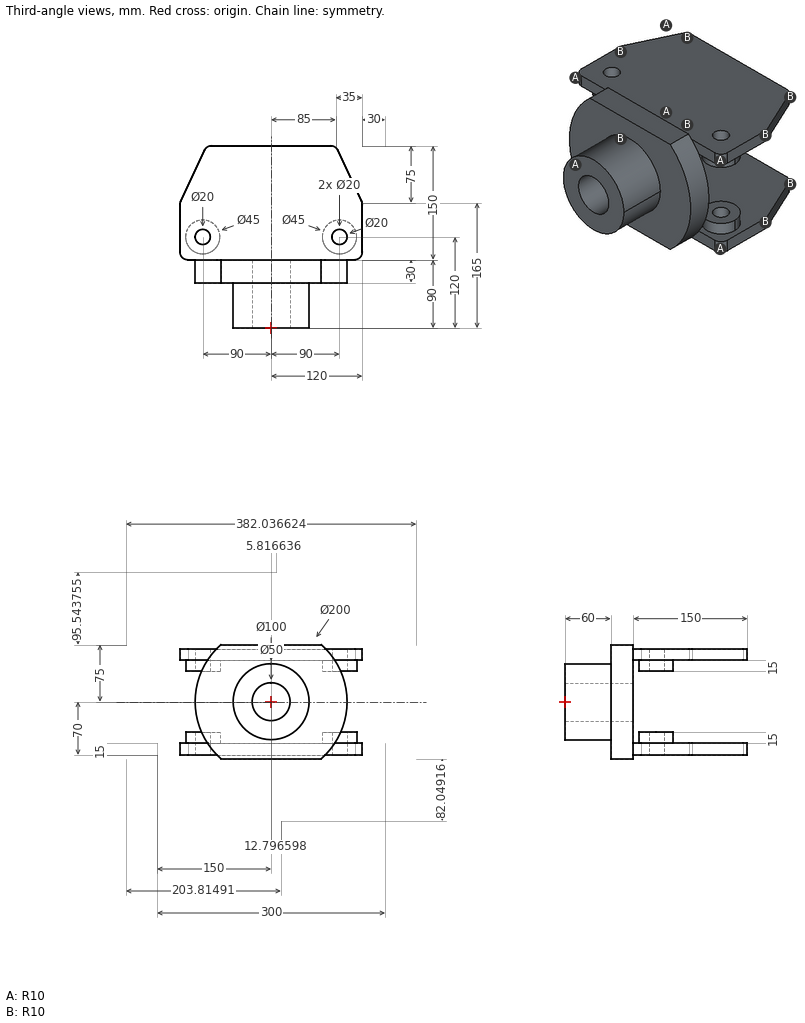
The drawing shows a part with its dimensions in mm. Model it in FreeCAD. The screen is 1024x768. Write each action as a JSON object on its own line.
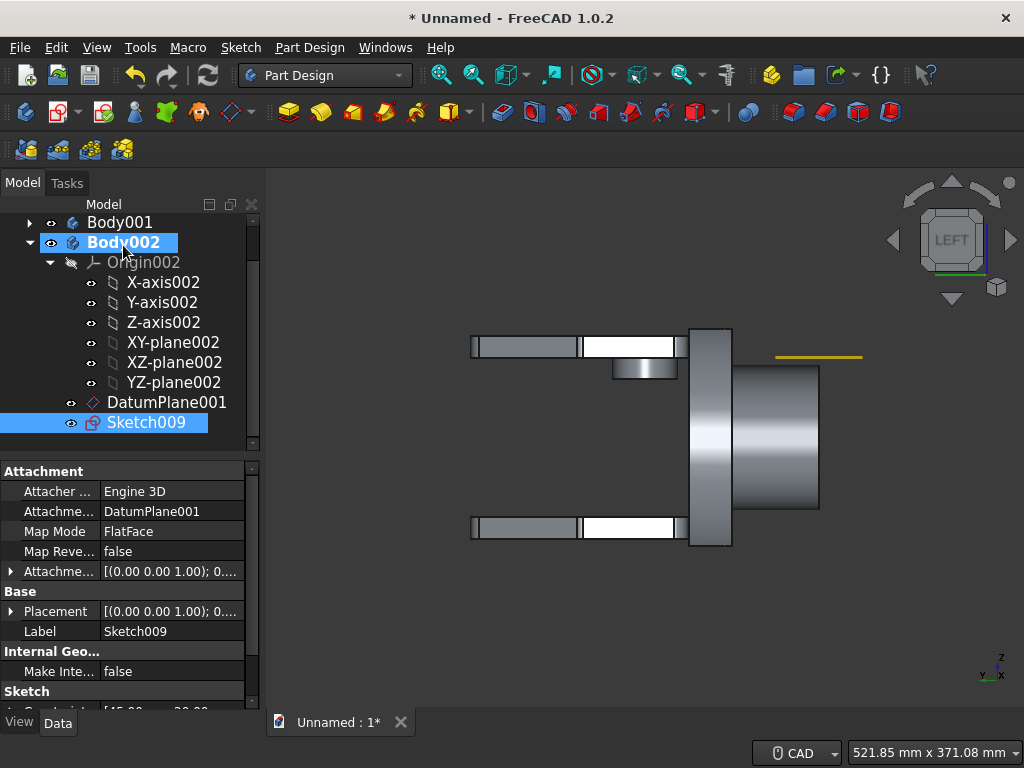
{"action": "left_click", "coordinate": [290, 112]}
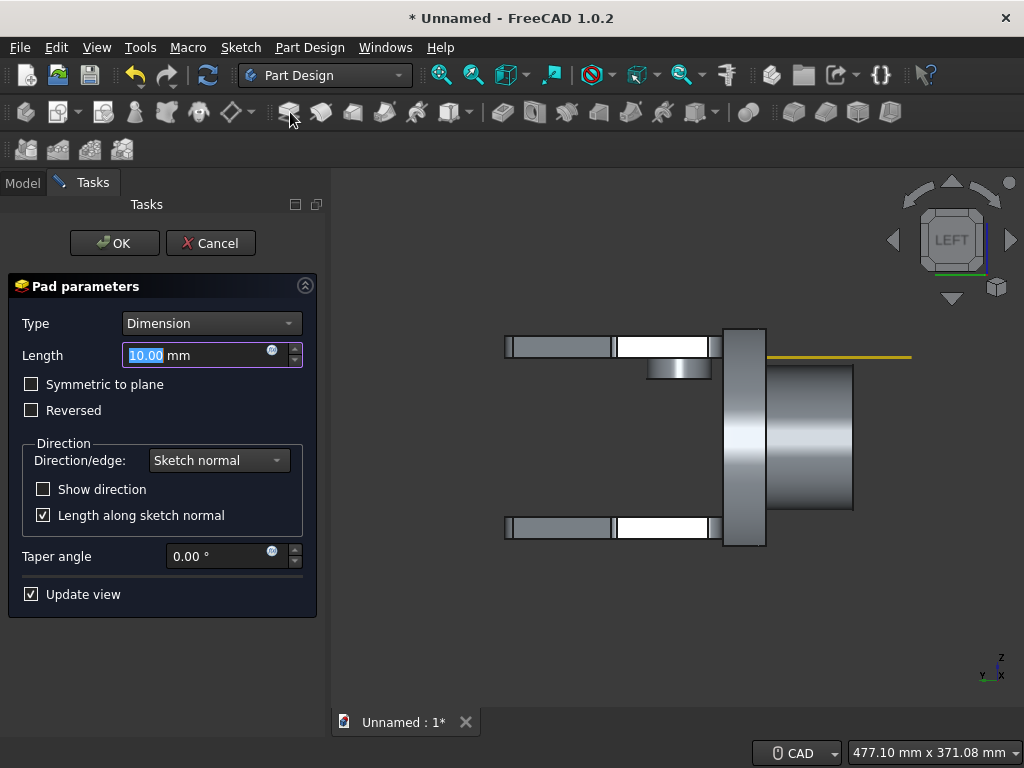
{"action": "type", "text": "15"}
{"action": "key", "text": "Tab"}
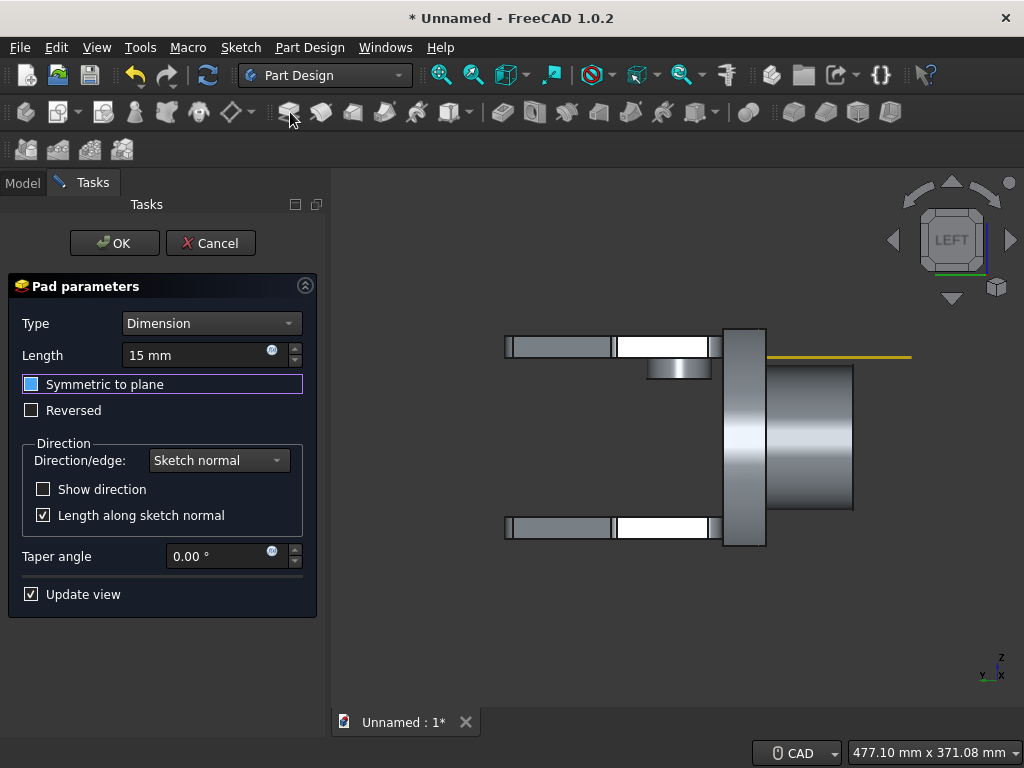
{"action": "left_click", "coordinate": [30, 410]}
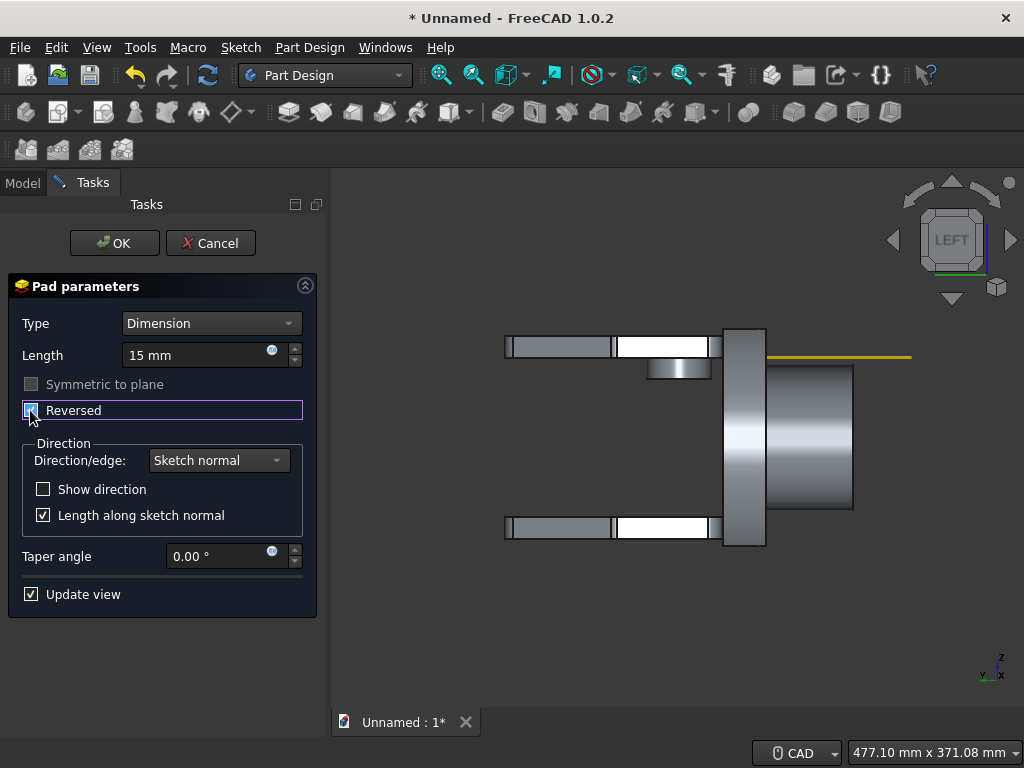
{"action": "left_click", "coordinate": [115, 243]}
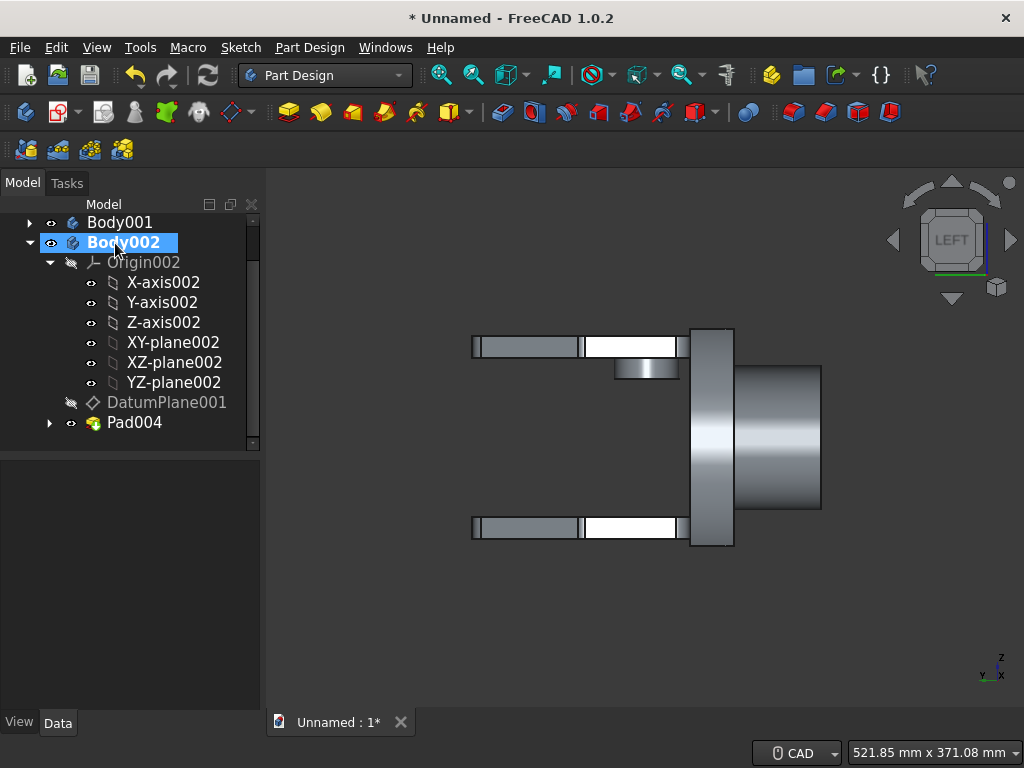
{"action": "left_click", "coordinate": [442, 76]}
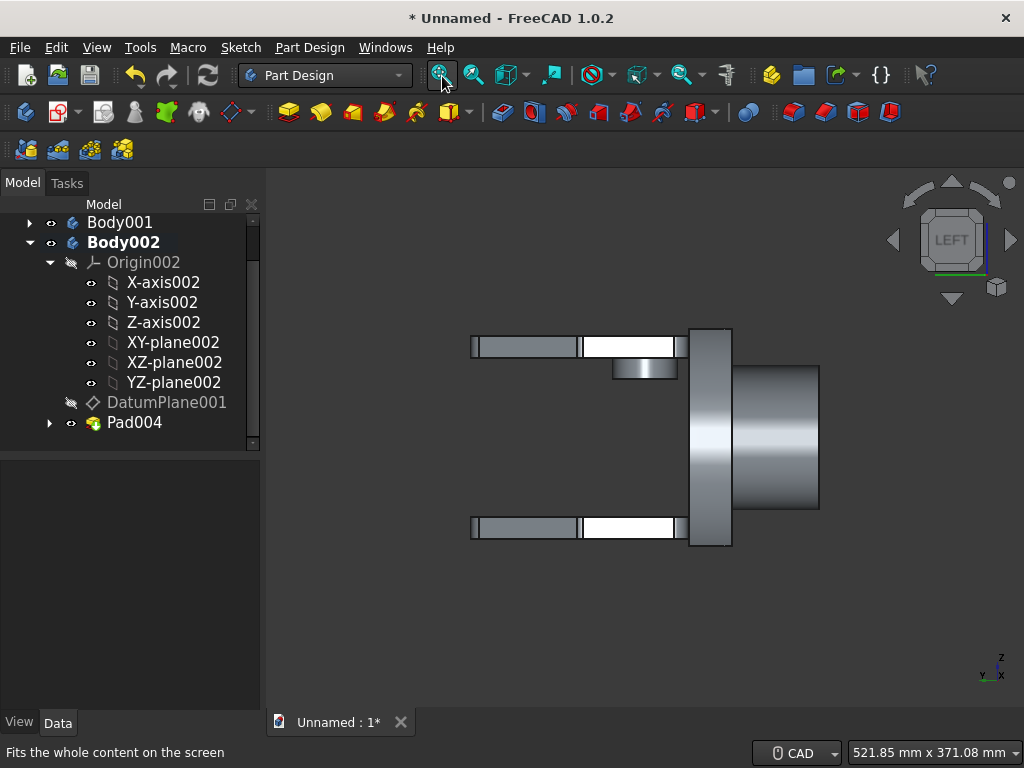
{"action": "left_click", "coordinate": [26, 112]}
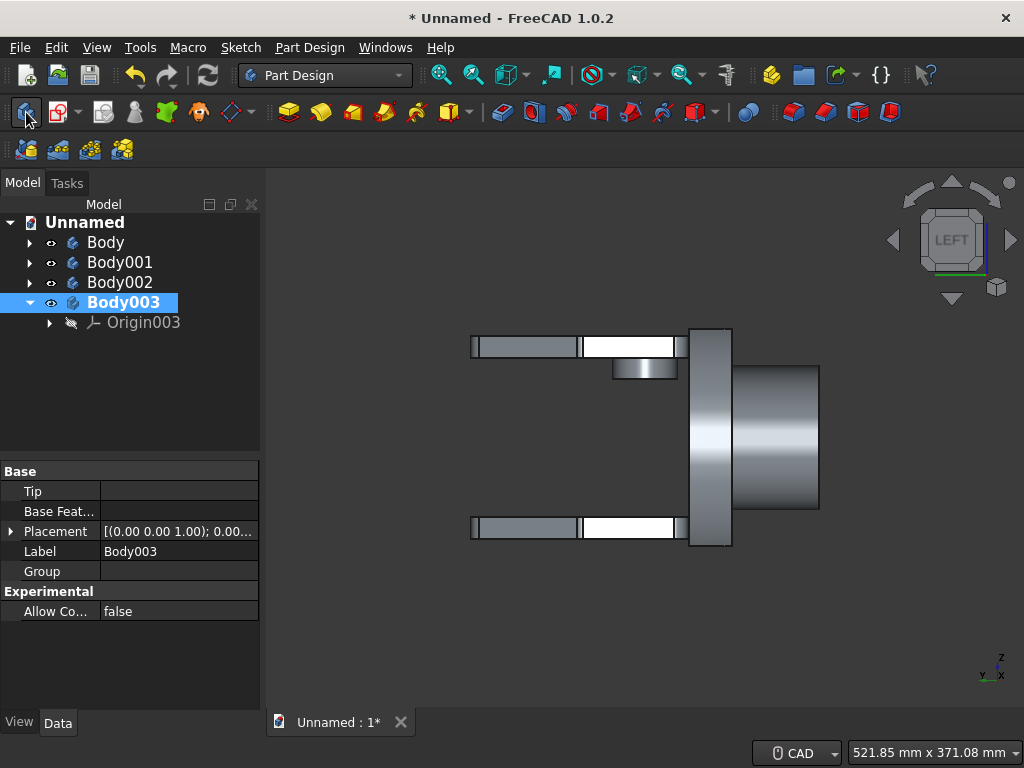
{"action": "left_click", "coordinate": [50, 323]}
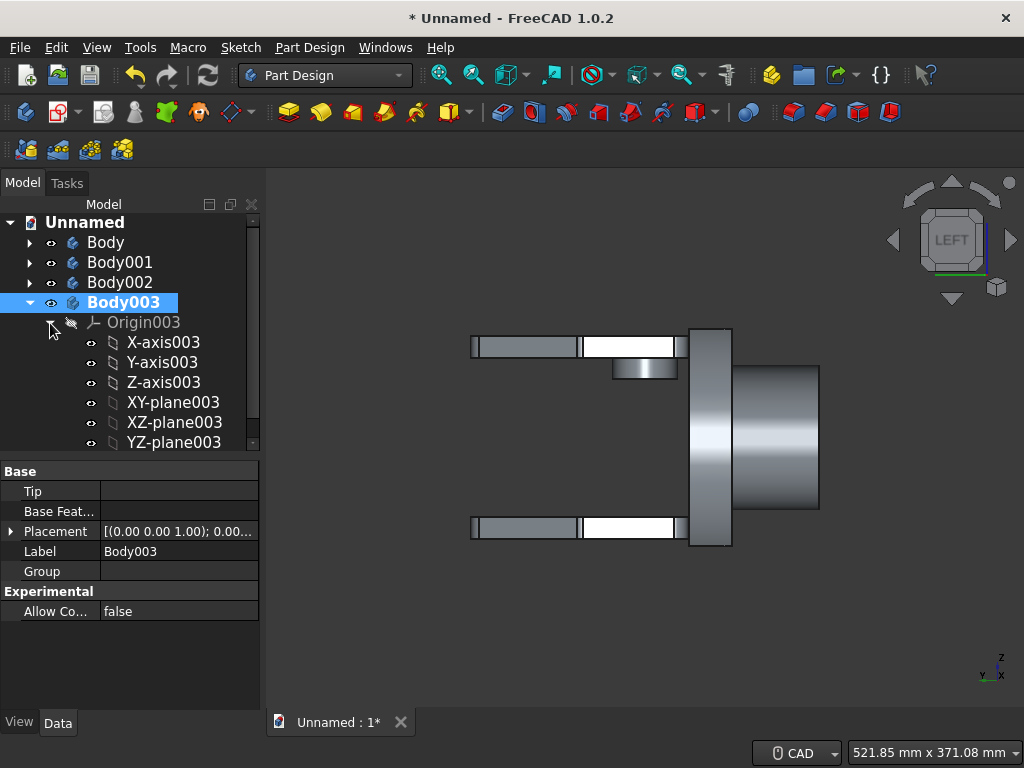
{"action": "left_click", "coordinate": [136, 403]}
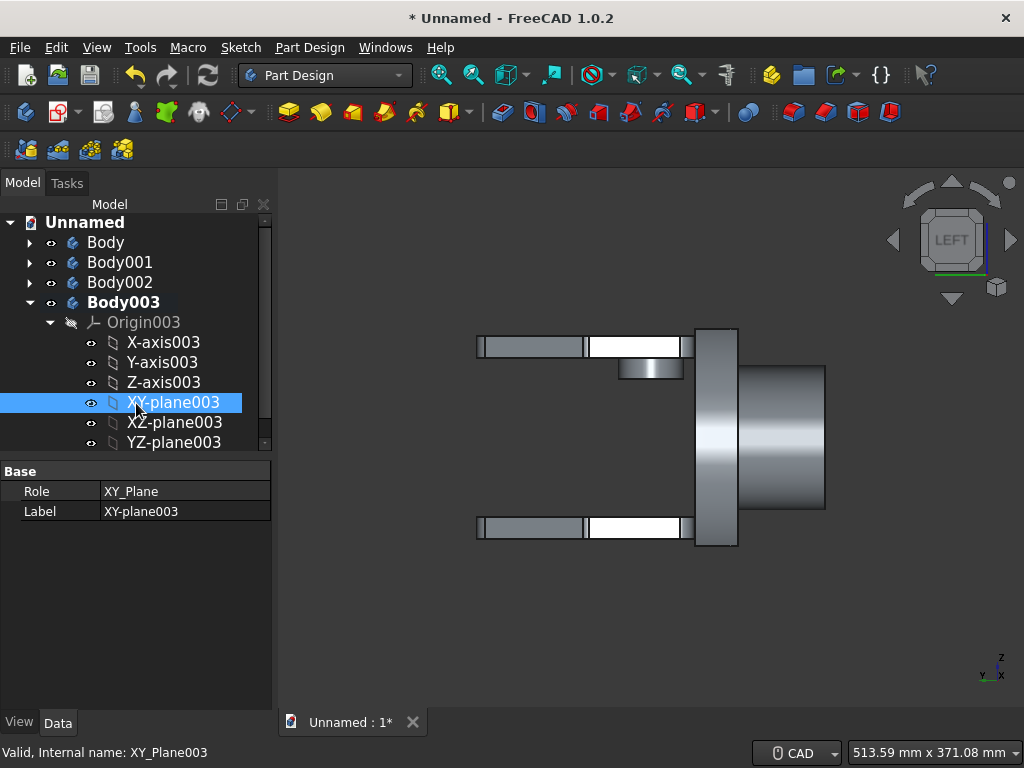
{"action": "left_click", "coordinate": [232, 112]}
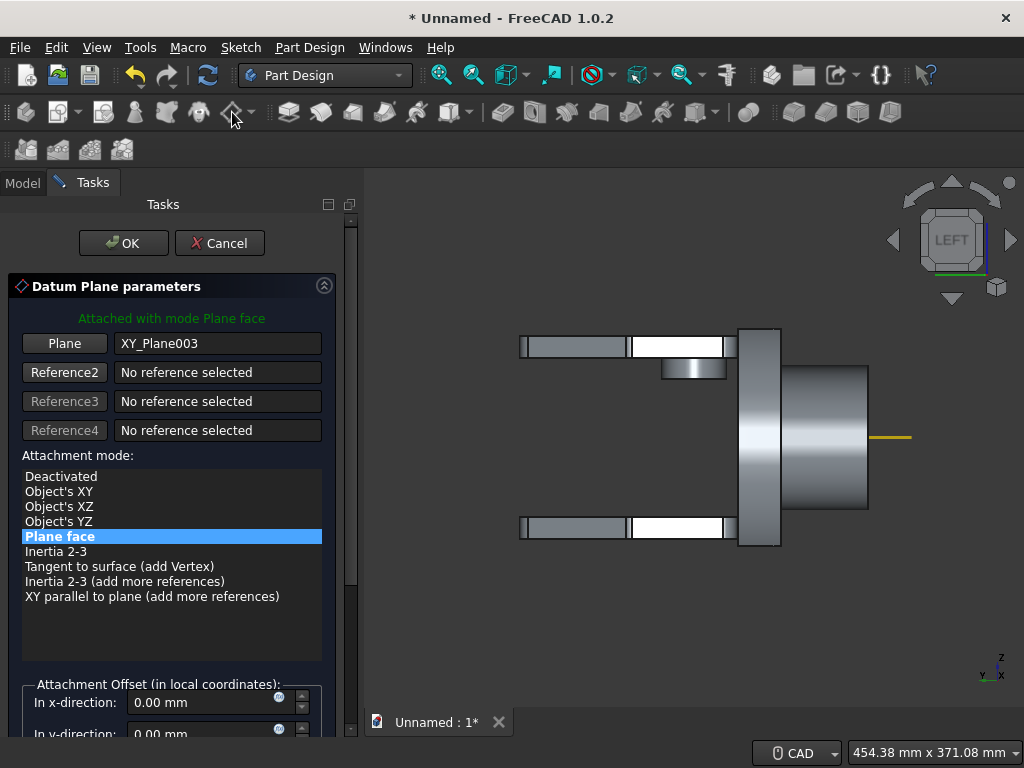
{"action": "scroll", "coordinate": [351, 475], "scroll_direction": "down", "scroll_amount": 2}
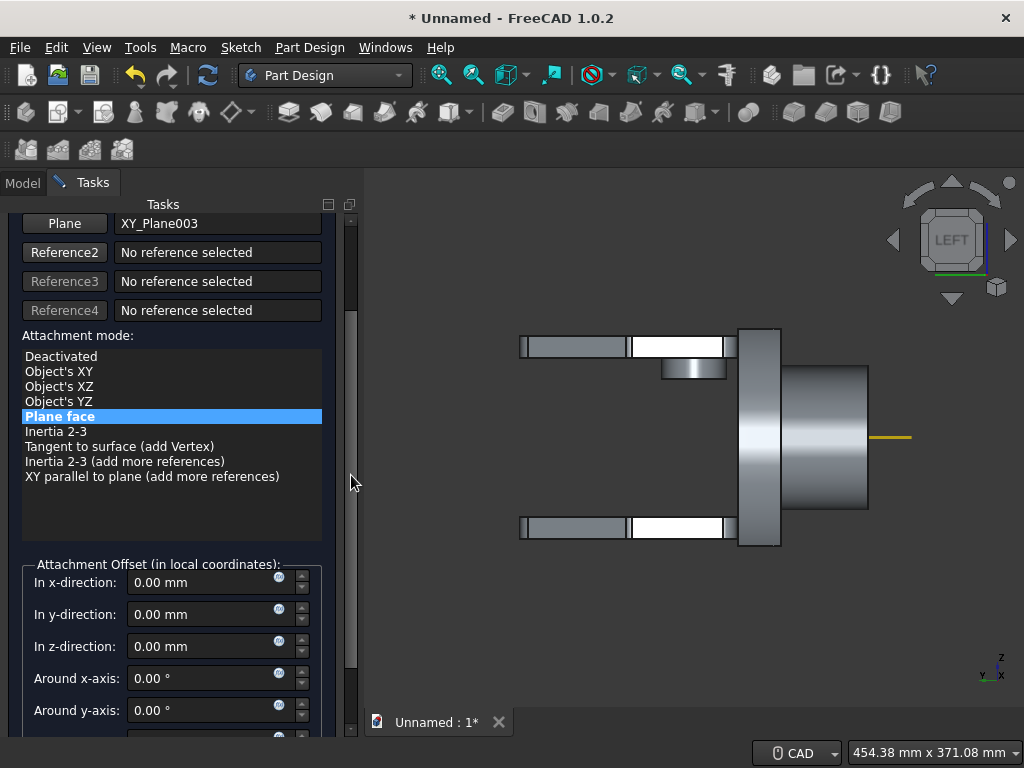
{"action": "triple_click", "coordinate": [210, 646]}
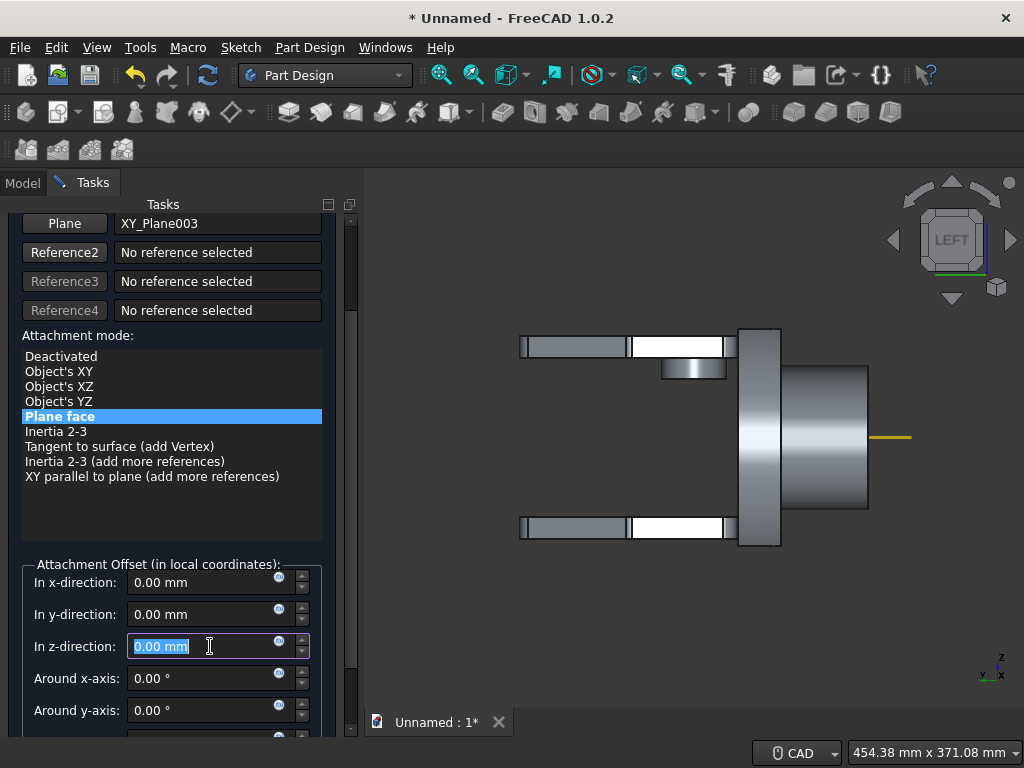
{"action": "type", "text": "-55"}
{"action": "key", "text": "Tab"}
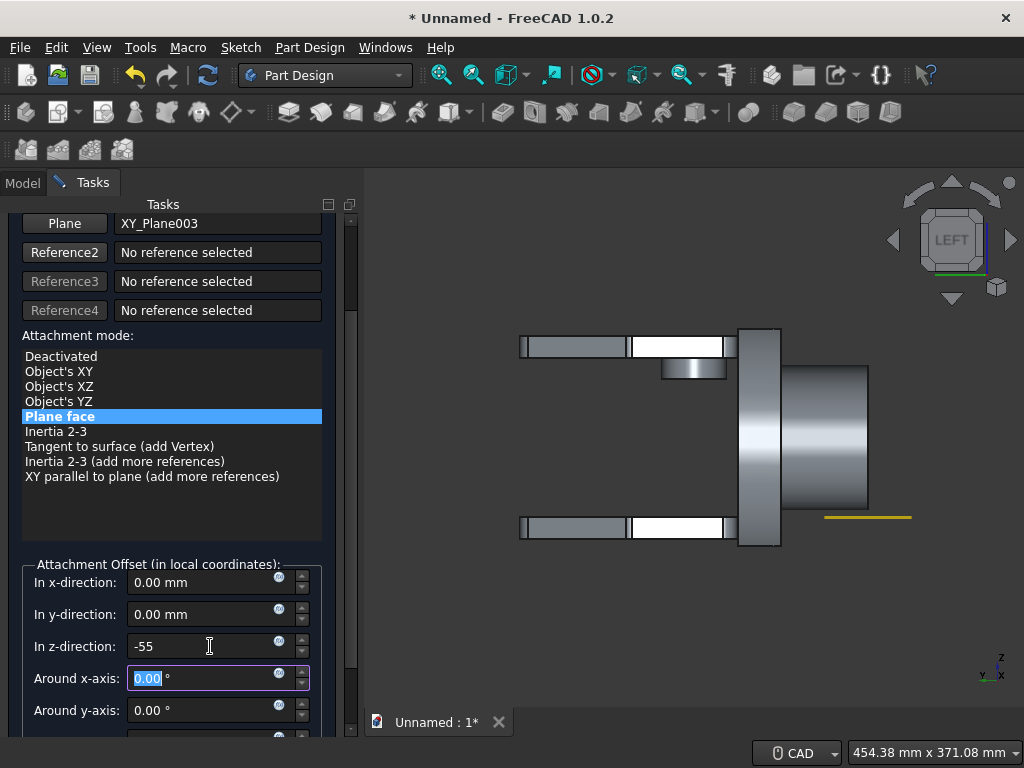
{"action": "scroll", "coordinate": [351, 475], "scroll_direction": "up", "scroll_amount": 3}